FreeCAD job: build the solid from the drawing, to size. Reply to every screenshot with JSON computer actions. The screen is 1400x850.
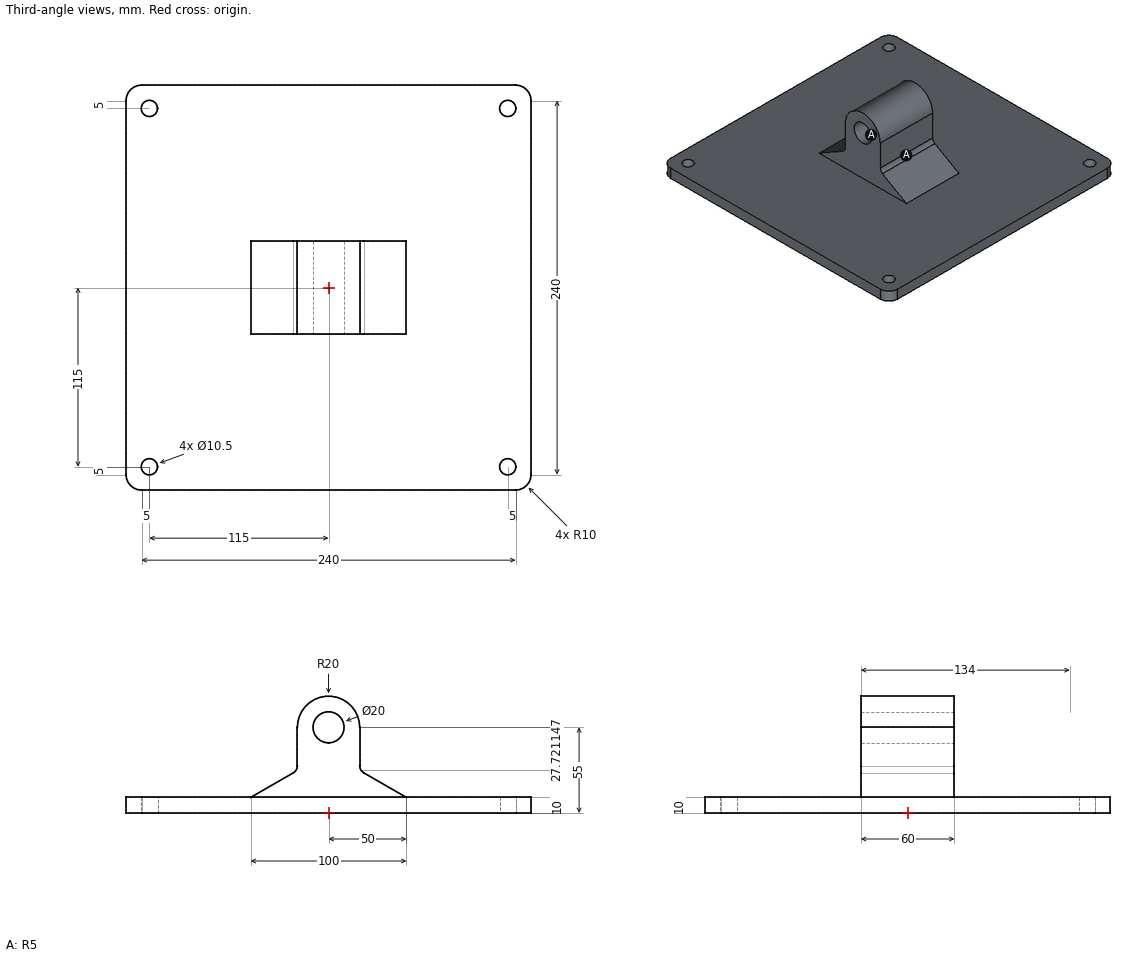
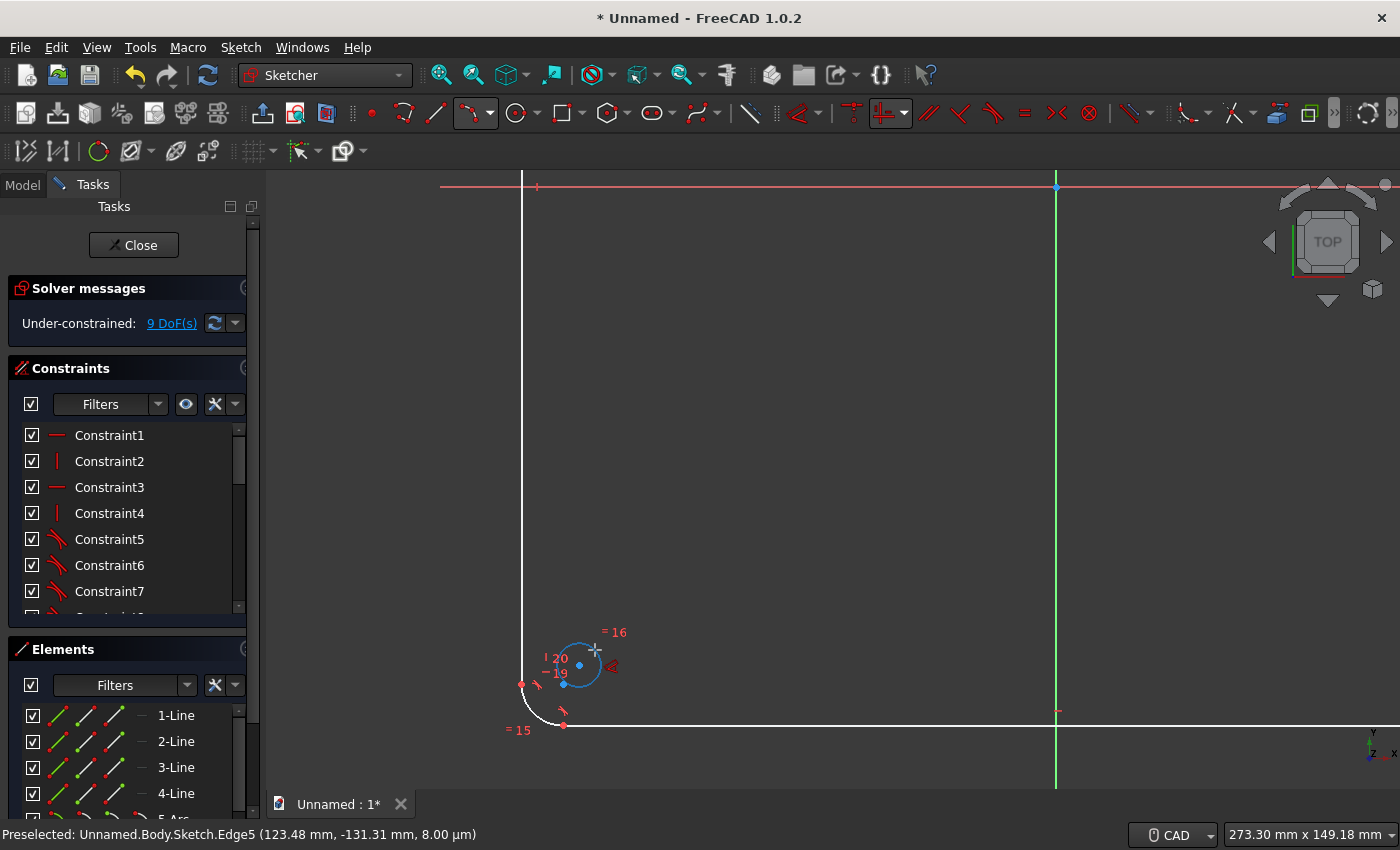
{"action": "left_click", "coordinate": [594, 650]}
{"action": "left_click", "coordinate": [616, 627]}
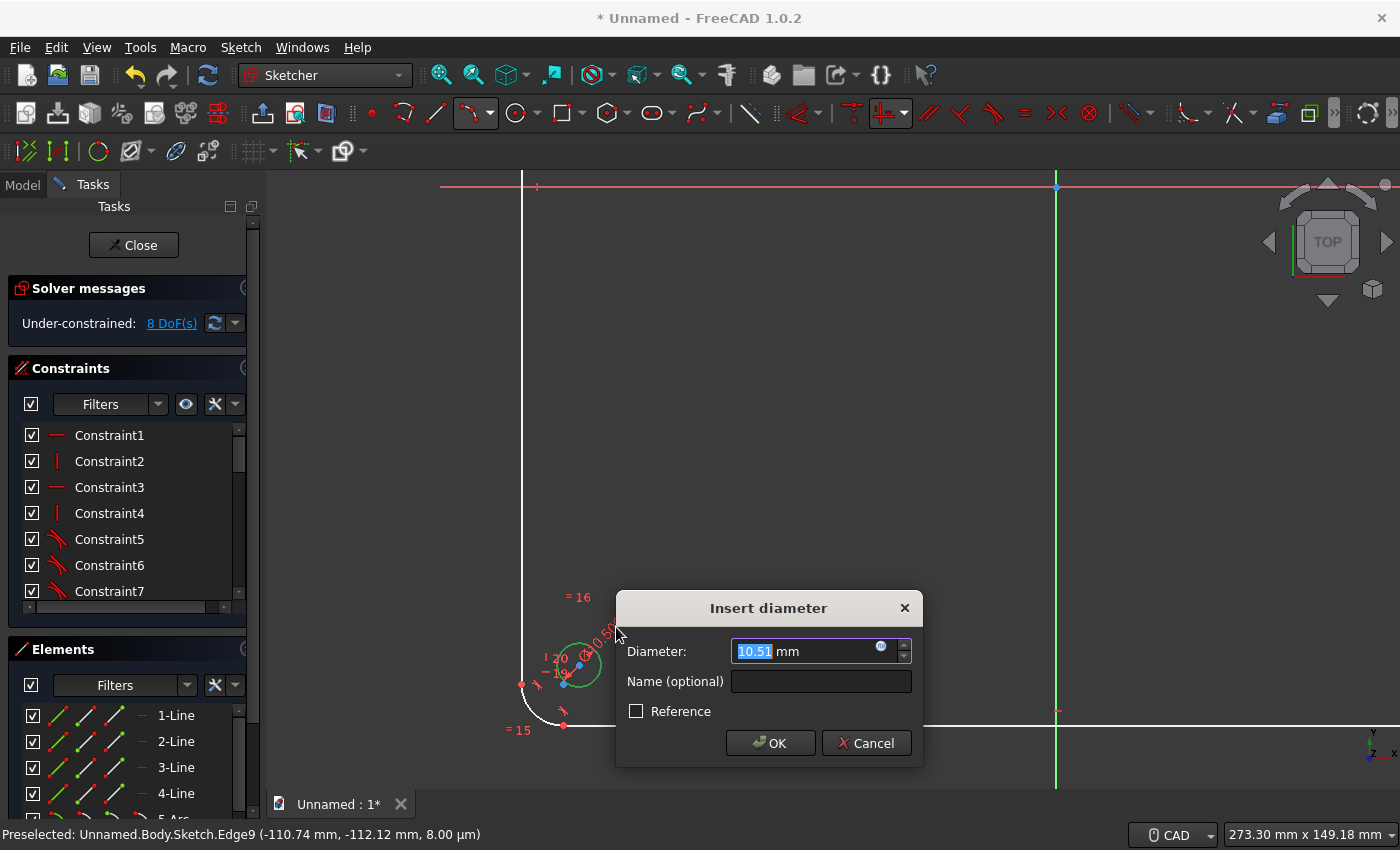
{"action": "type", "text": "10.5"}
{"action": "key", "text": "Return"}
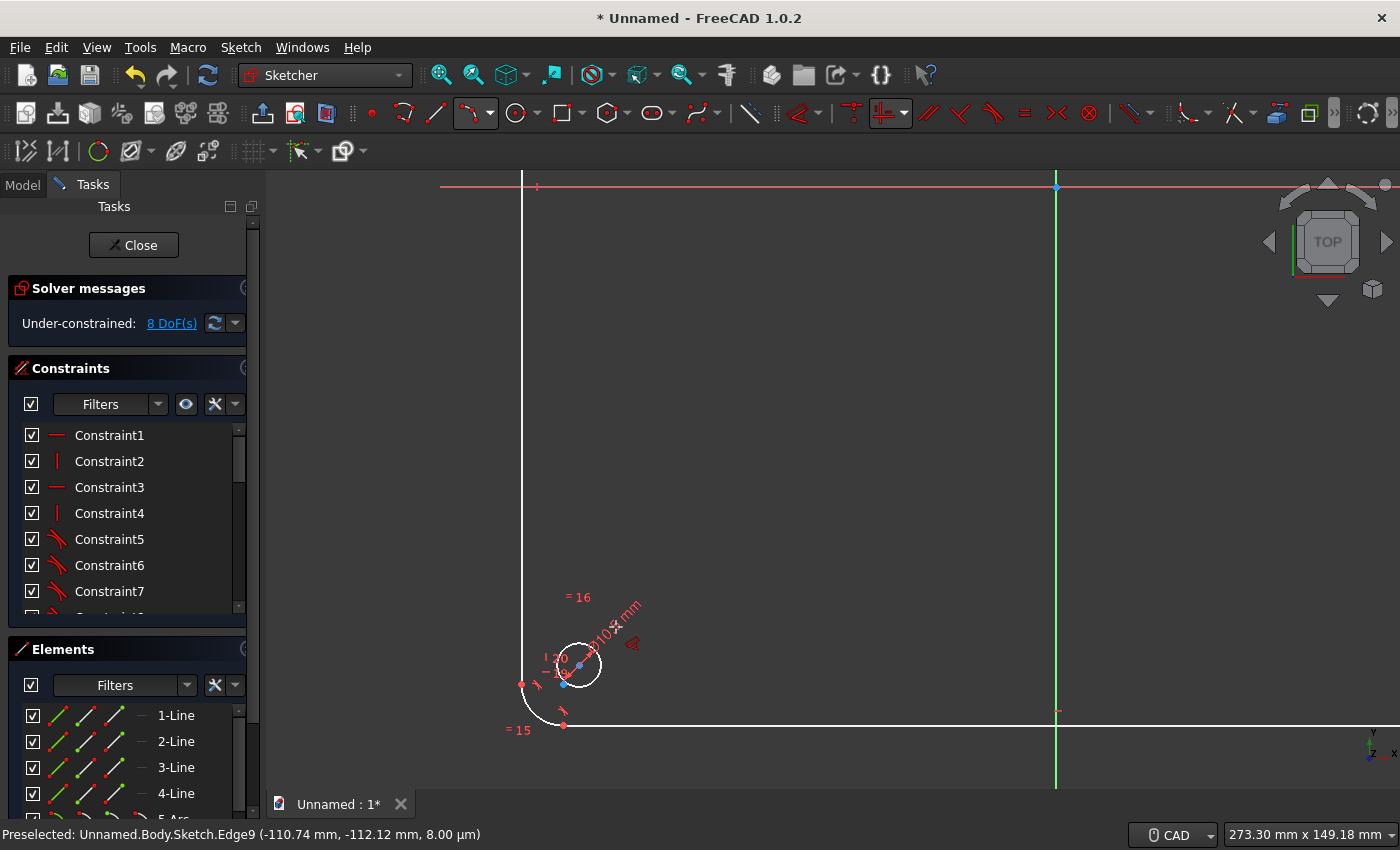
{"action": "scroll", "coordinate": [563, 726], "scroll_direction": "up", "scroll_amount": 4}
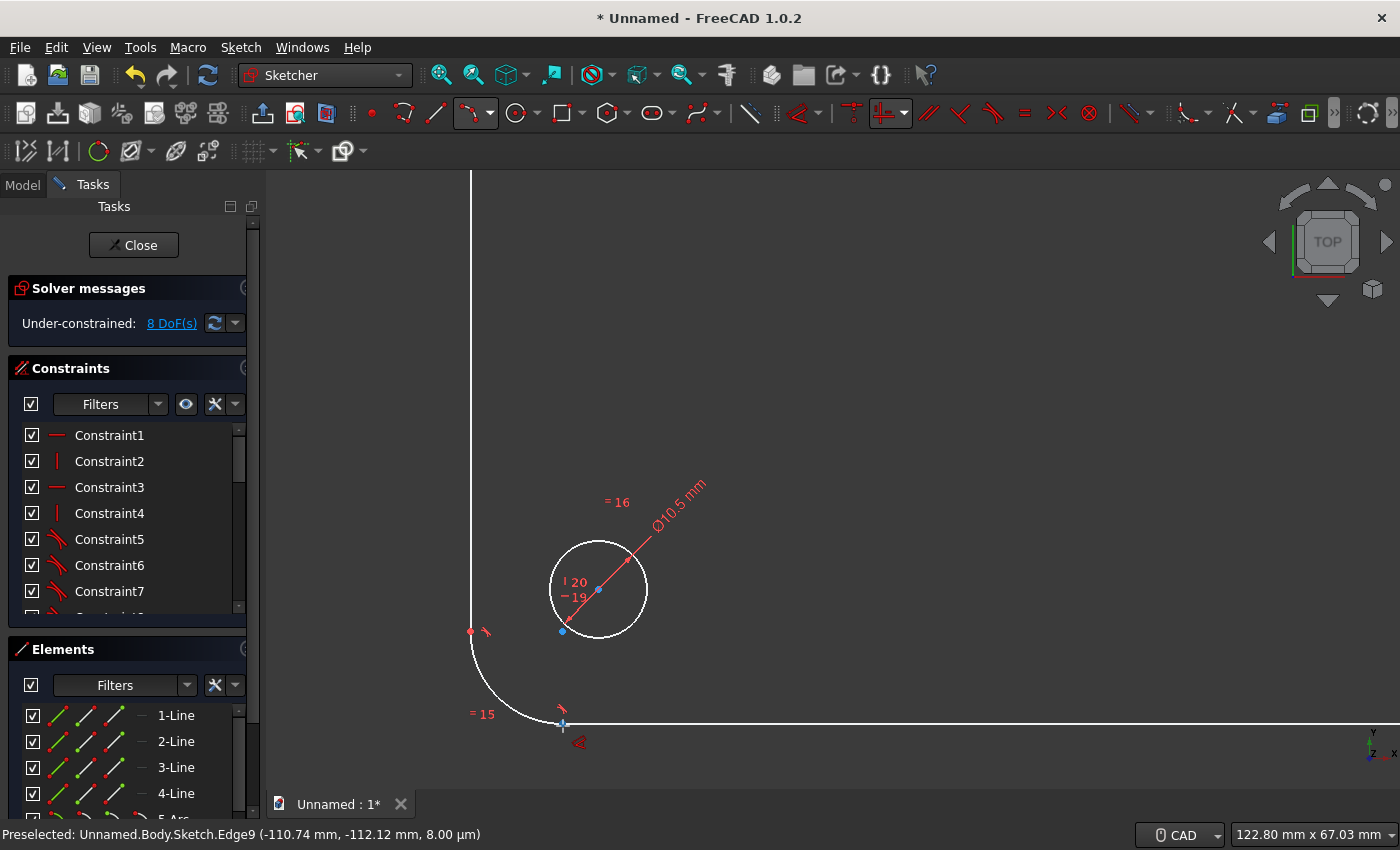
{"action": "left_click", "coordinate": [563, 724]}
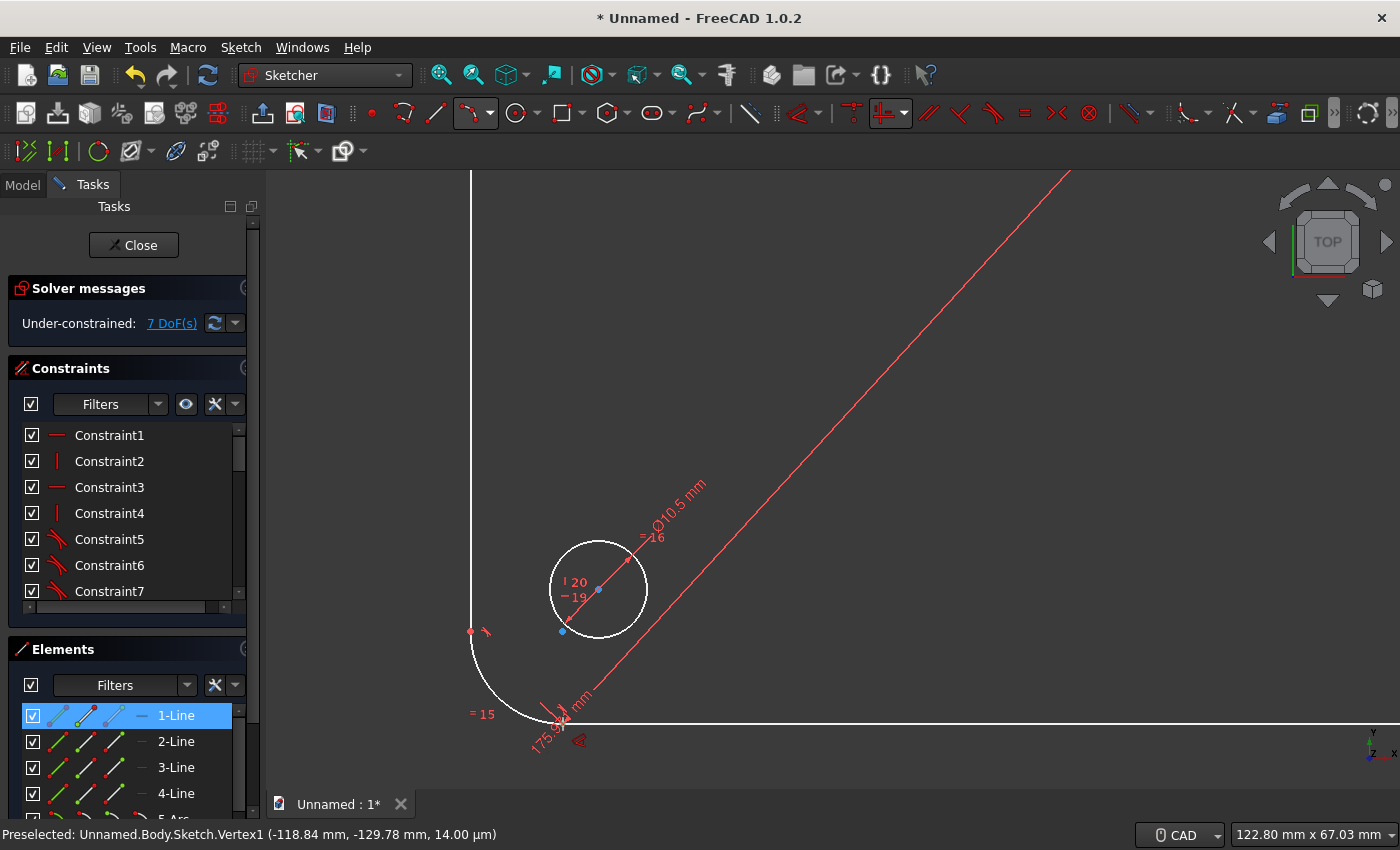
{"action": "left_click", "coordinate": [598, 589]}
{"action": "left_click", "coordinate": [581, 758]}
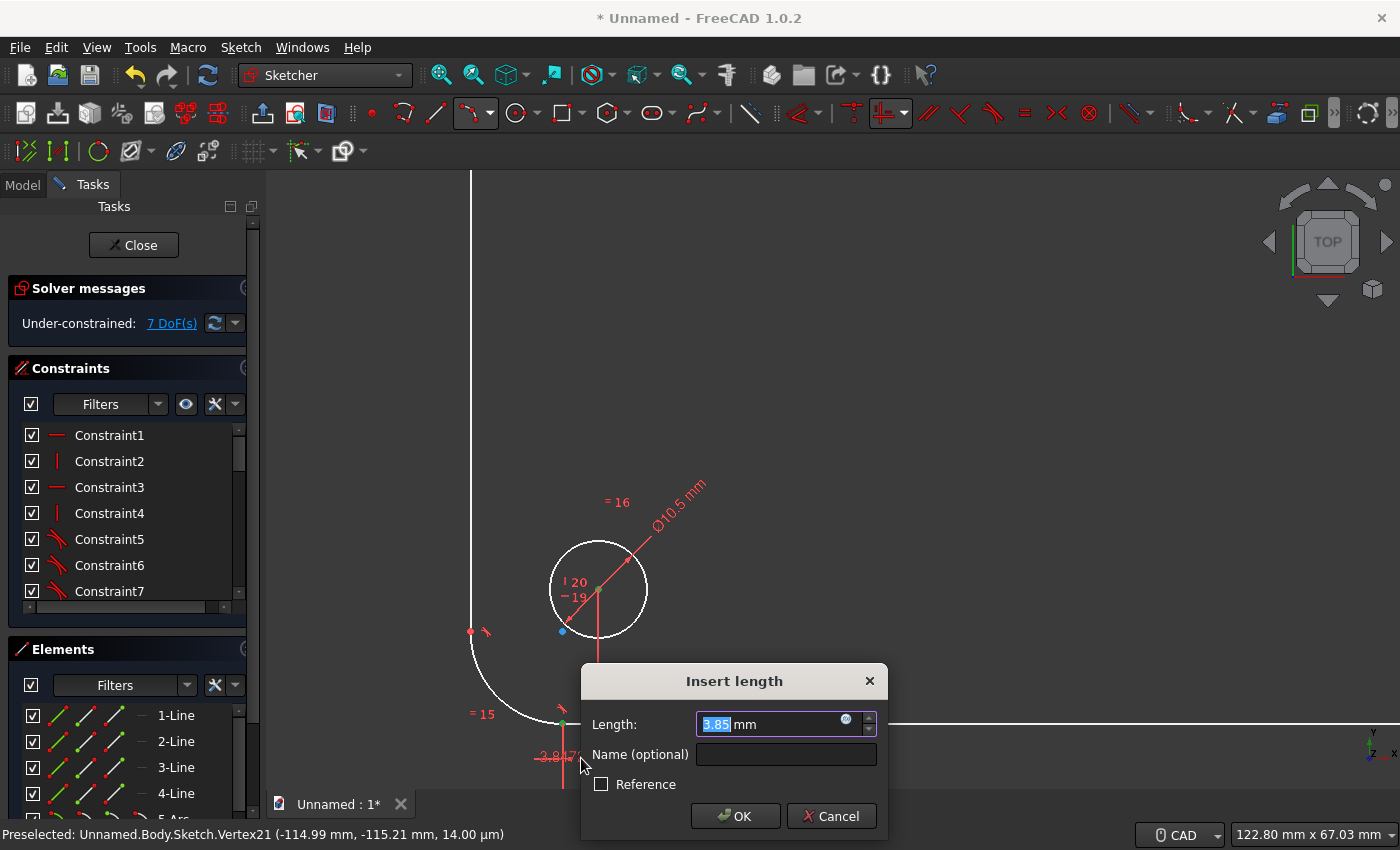
{"action": "type", "text": "5"}
{"action": "key", "text": "Return"}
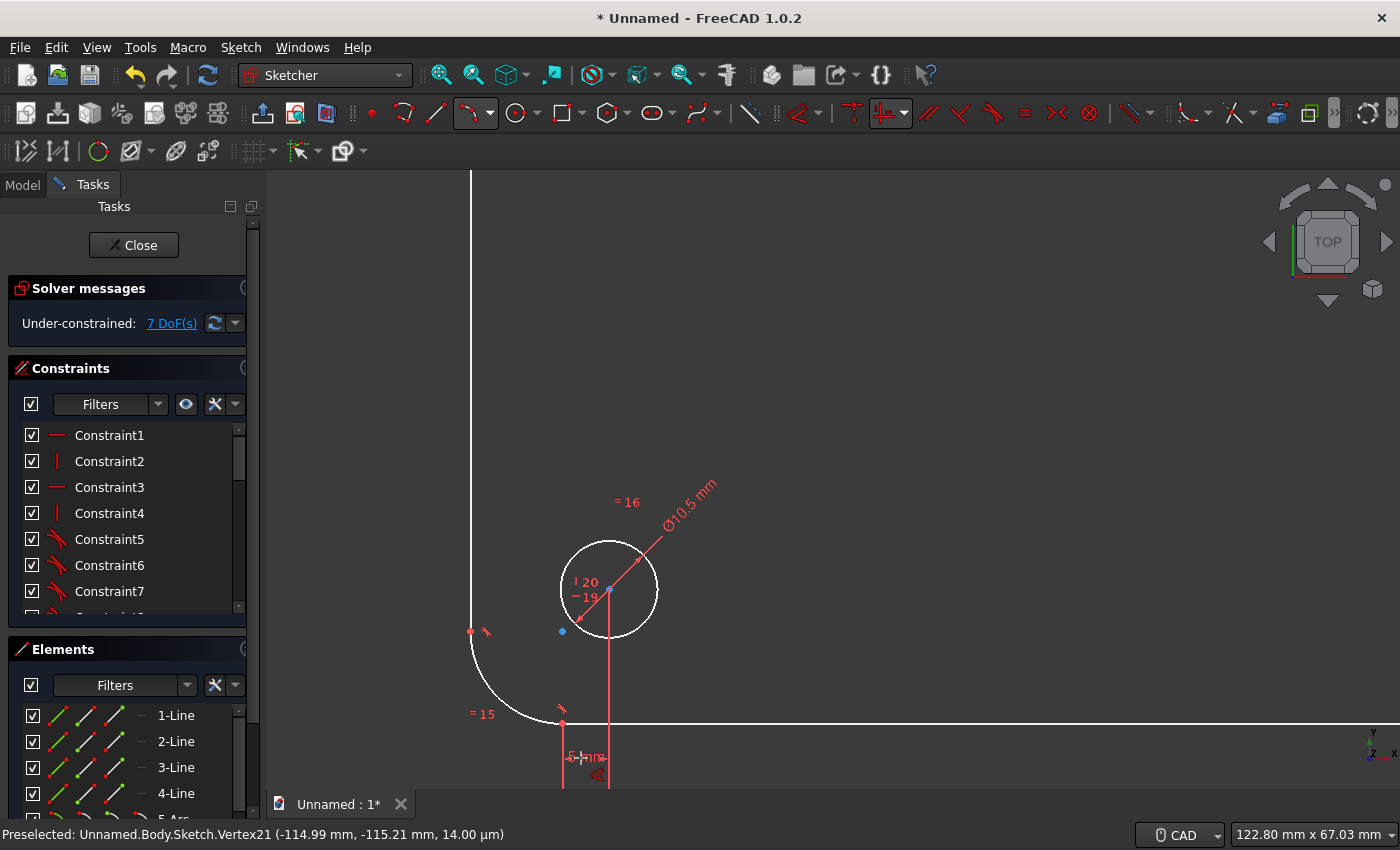
{"action": "left_click", "coordinate": [471, 632]}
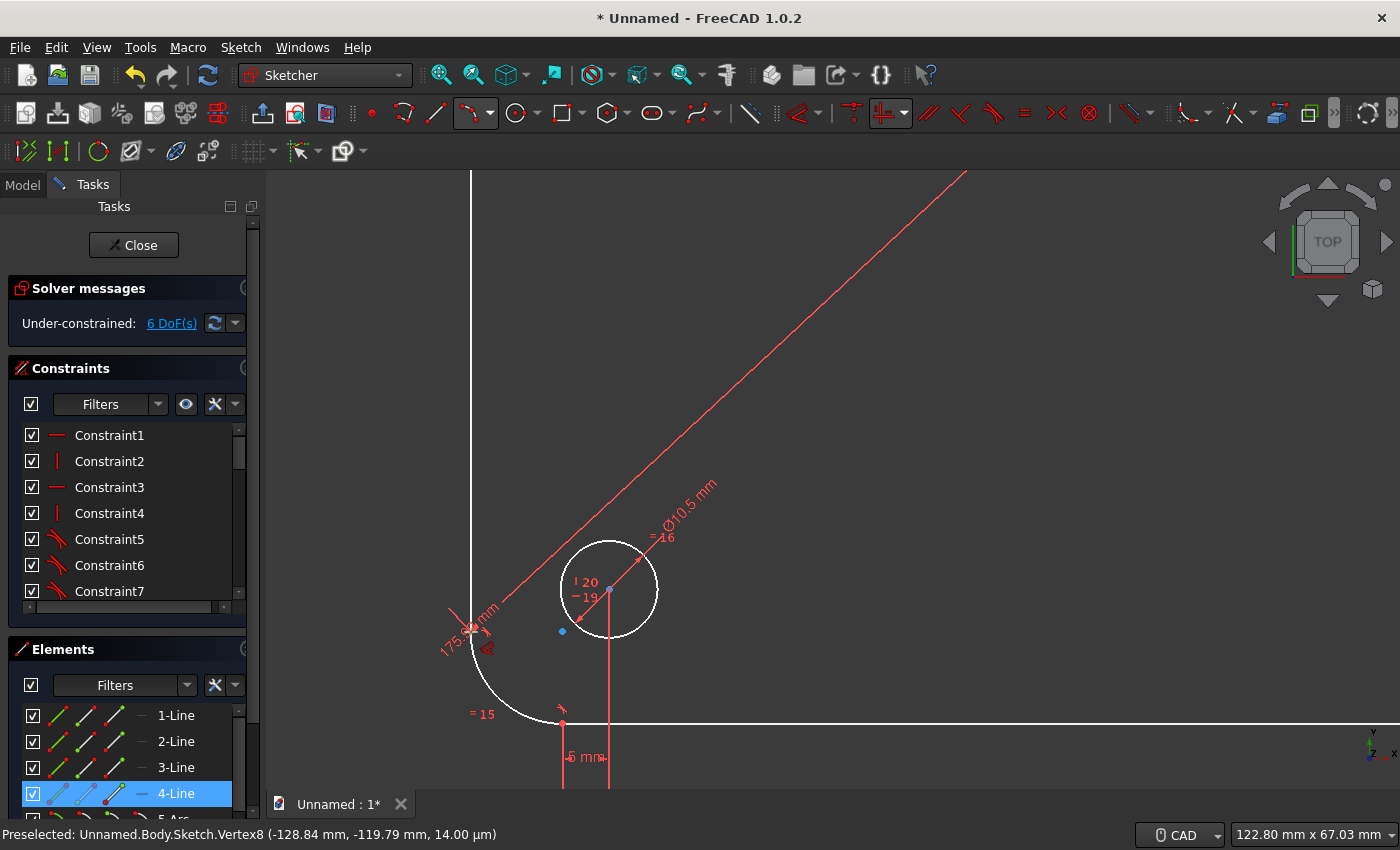
{"action": "left_click", "coordinate": [609, 589]}
{"action": "left_click", "coordinate": [437, 611]}